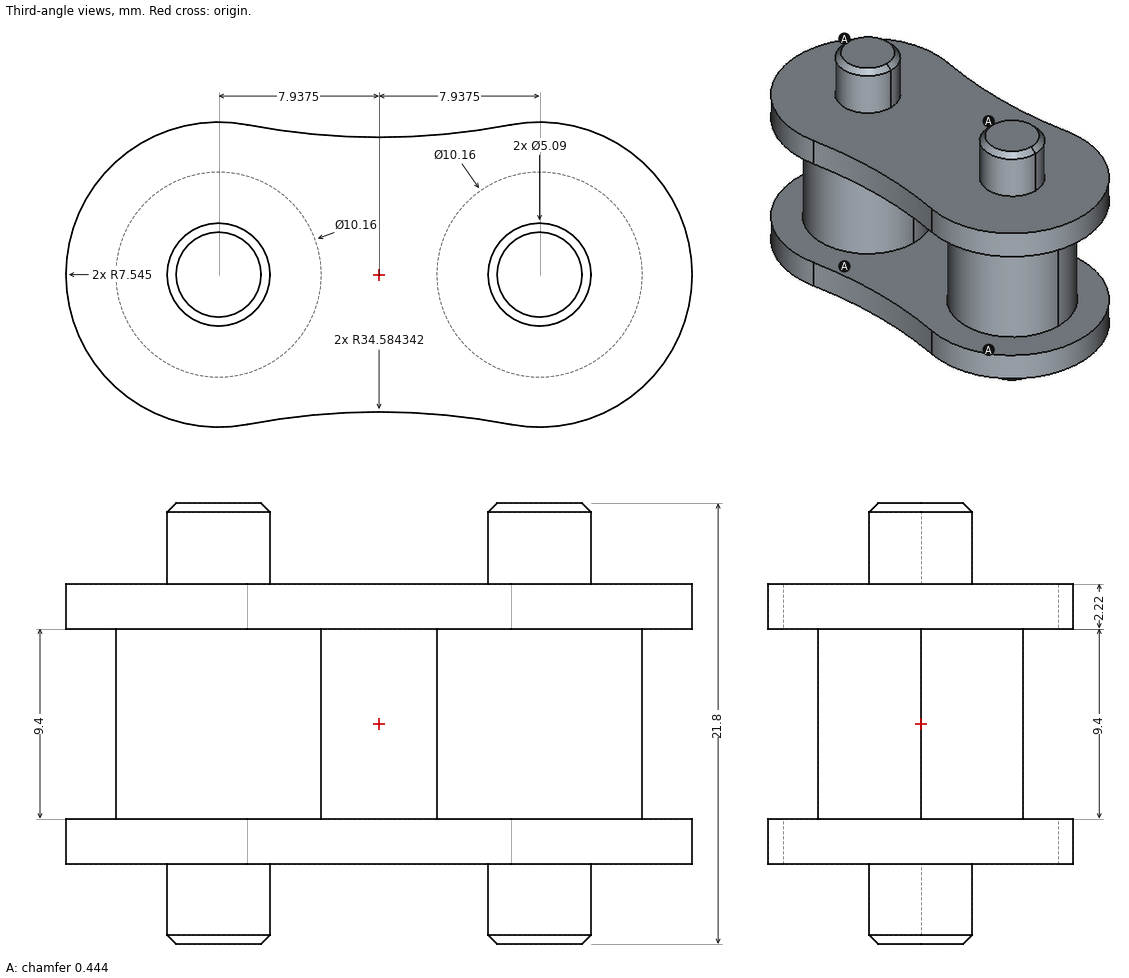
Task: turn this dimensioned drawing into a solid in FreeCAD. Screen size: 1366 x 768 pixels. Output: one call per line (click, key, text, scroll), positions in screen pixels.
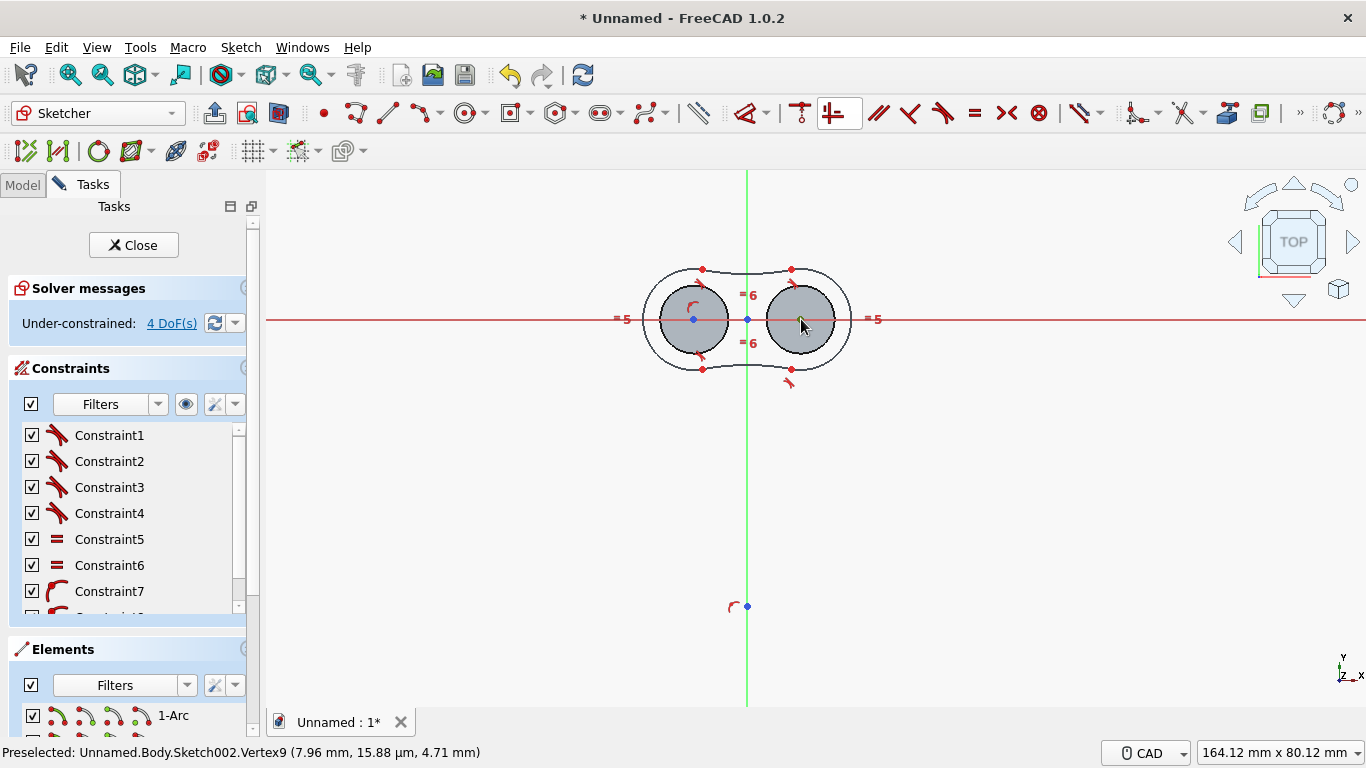
click(359, 320)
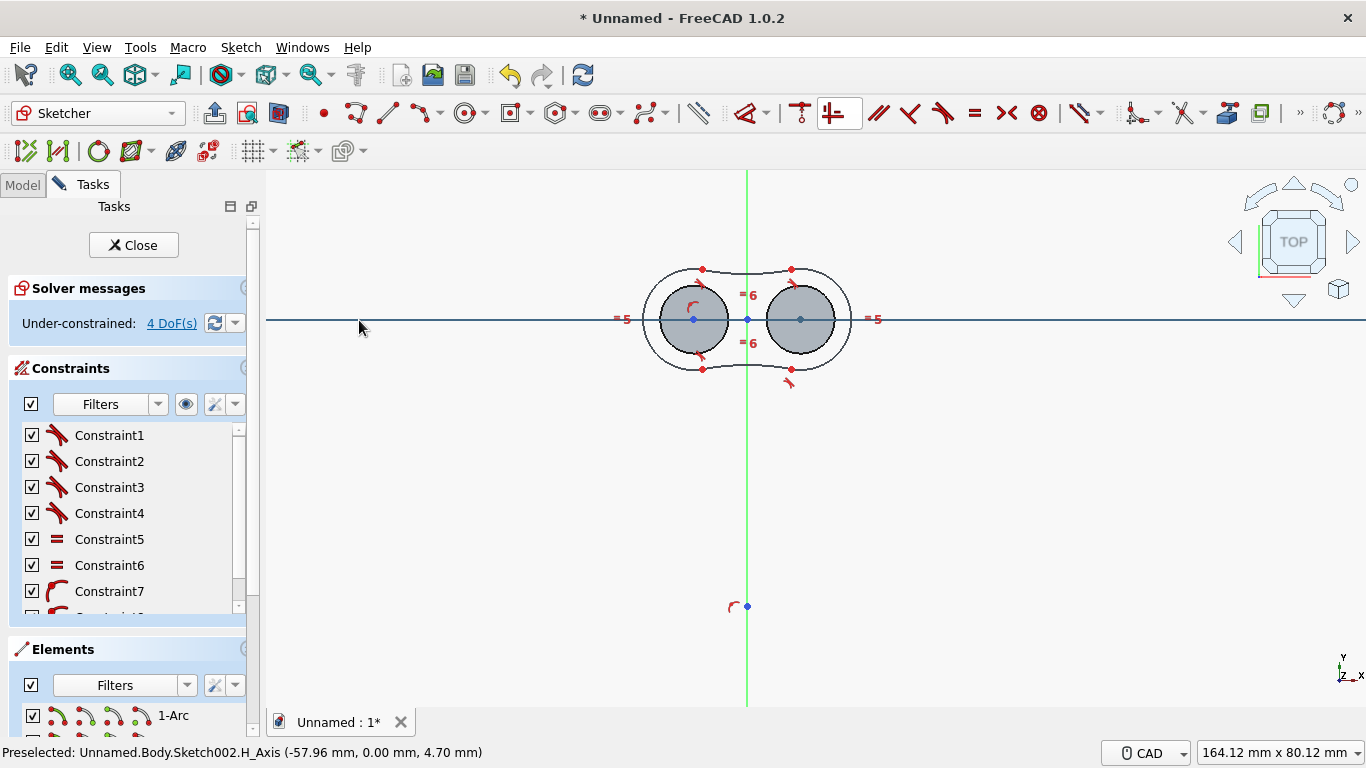
key(c)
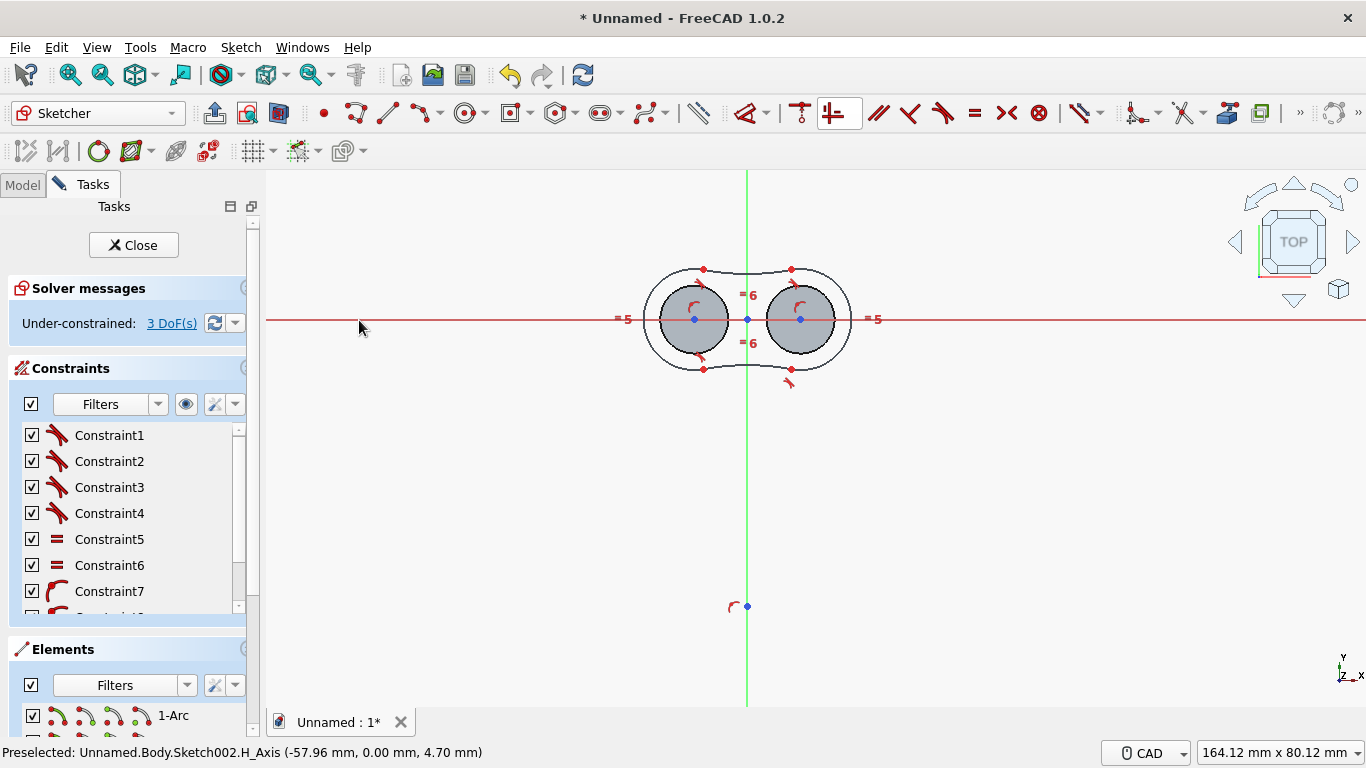
click(746, 114)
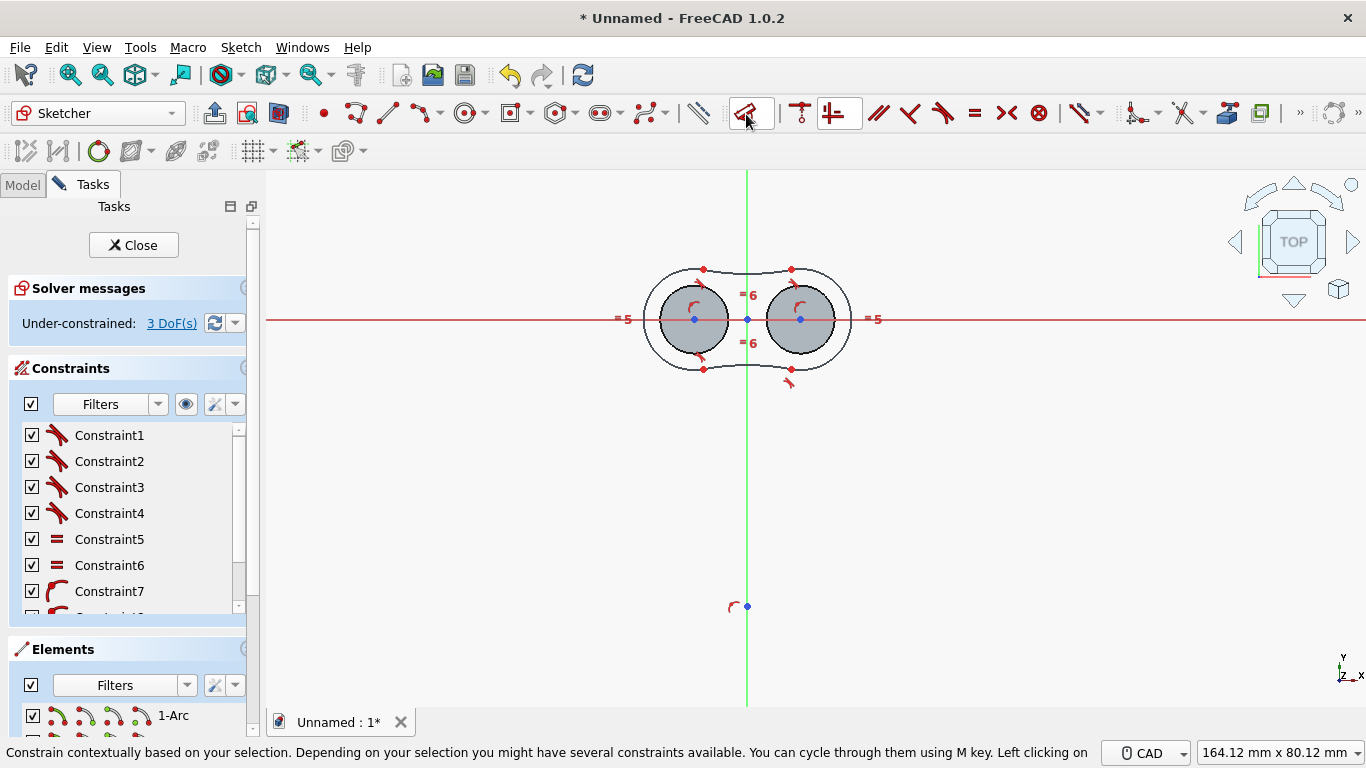
click(656, 287)
click(632, 266)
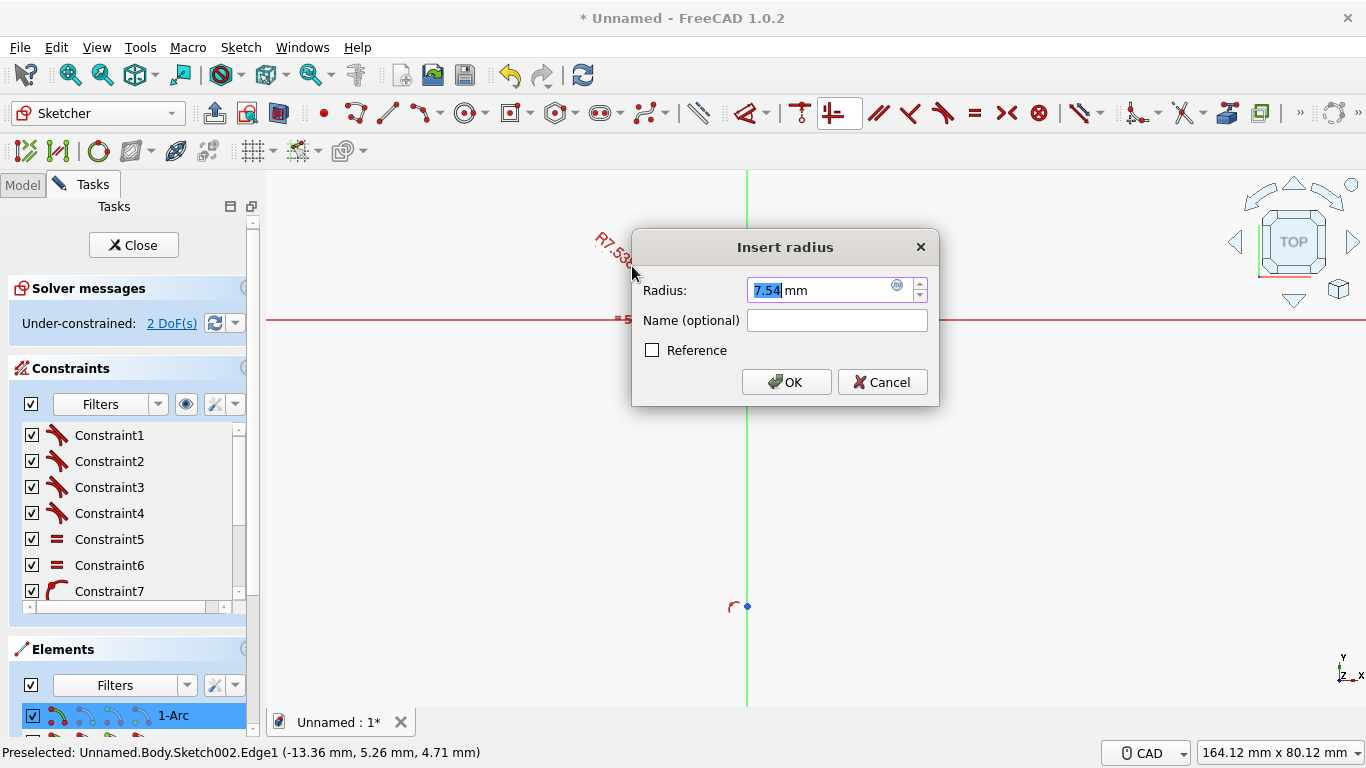
text(7.545)
key(Return)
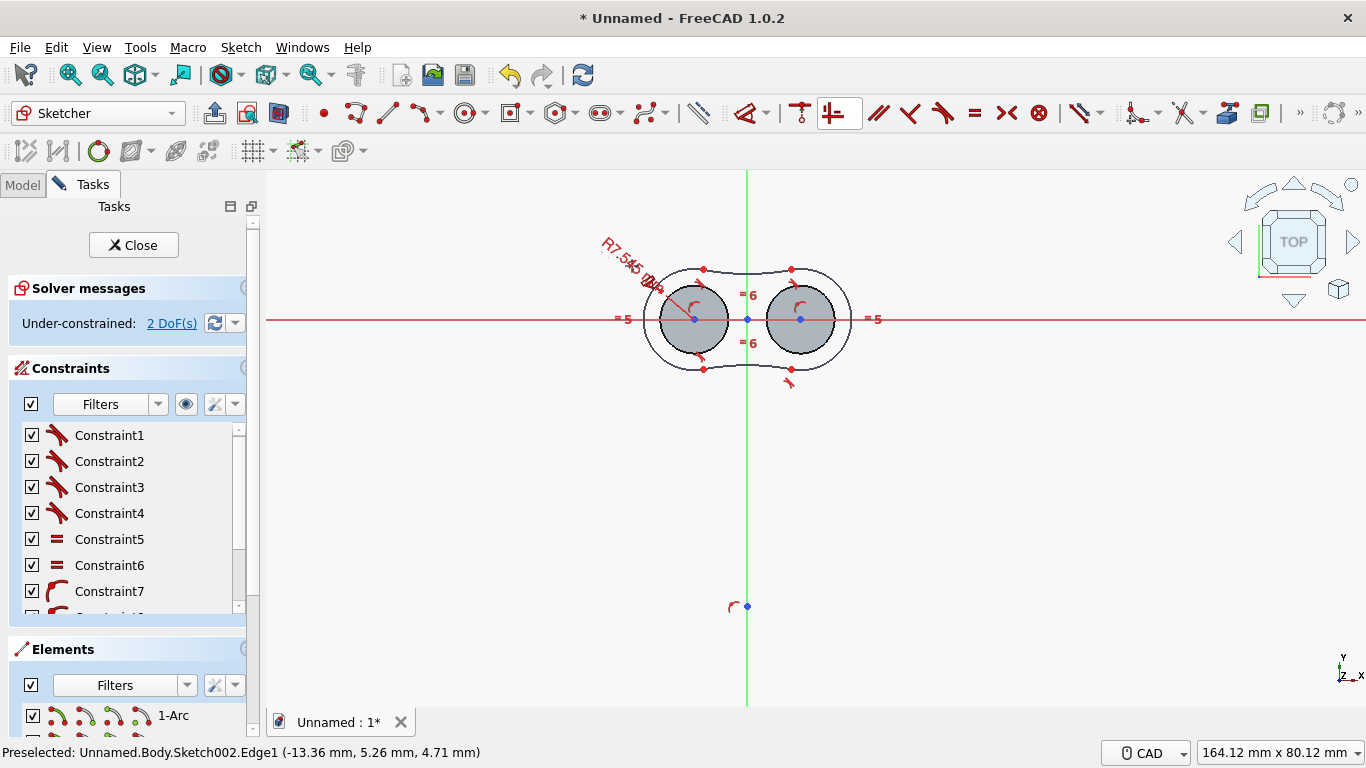
click(765, 366)
click(767, 334)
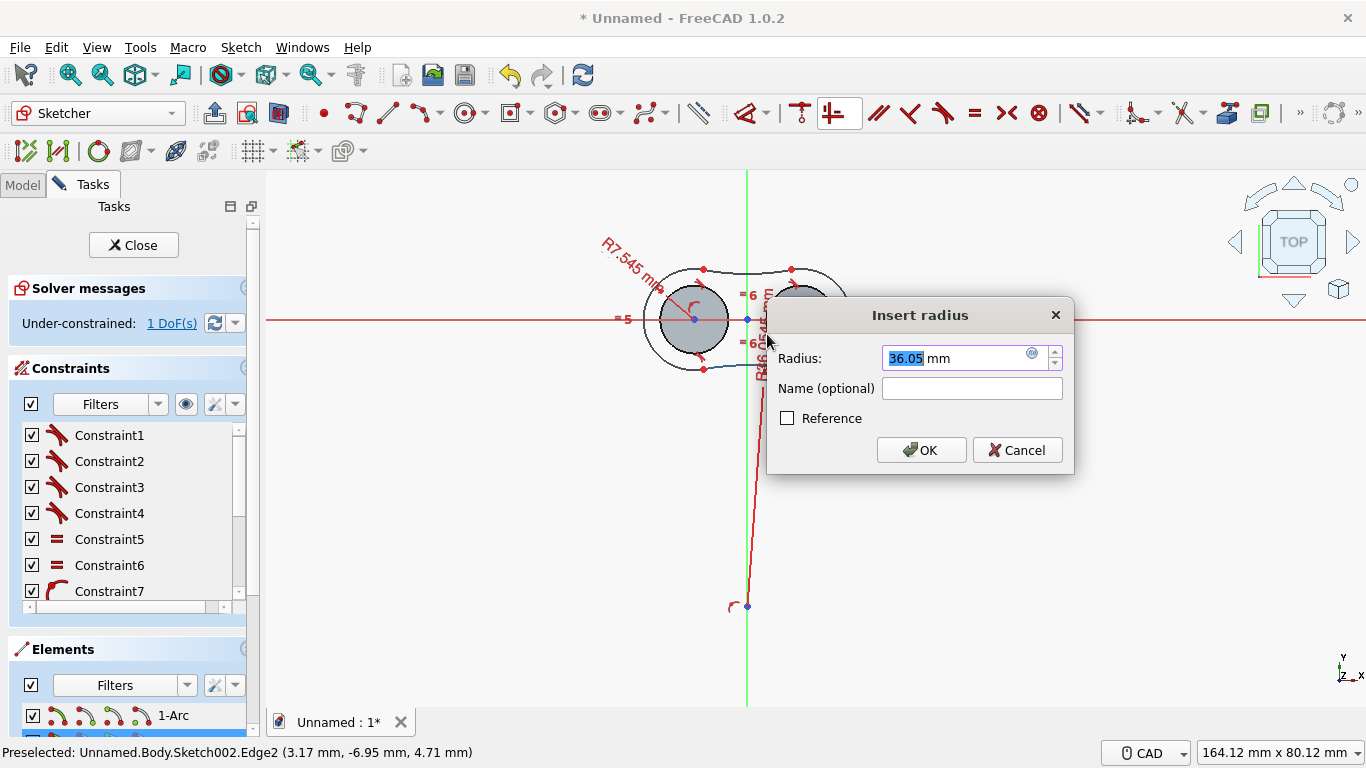
text(34.584342)
key(Return)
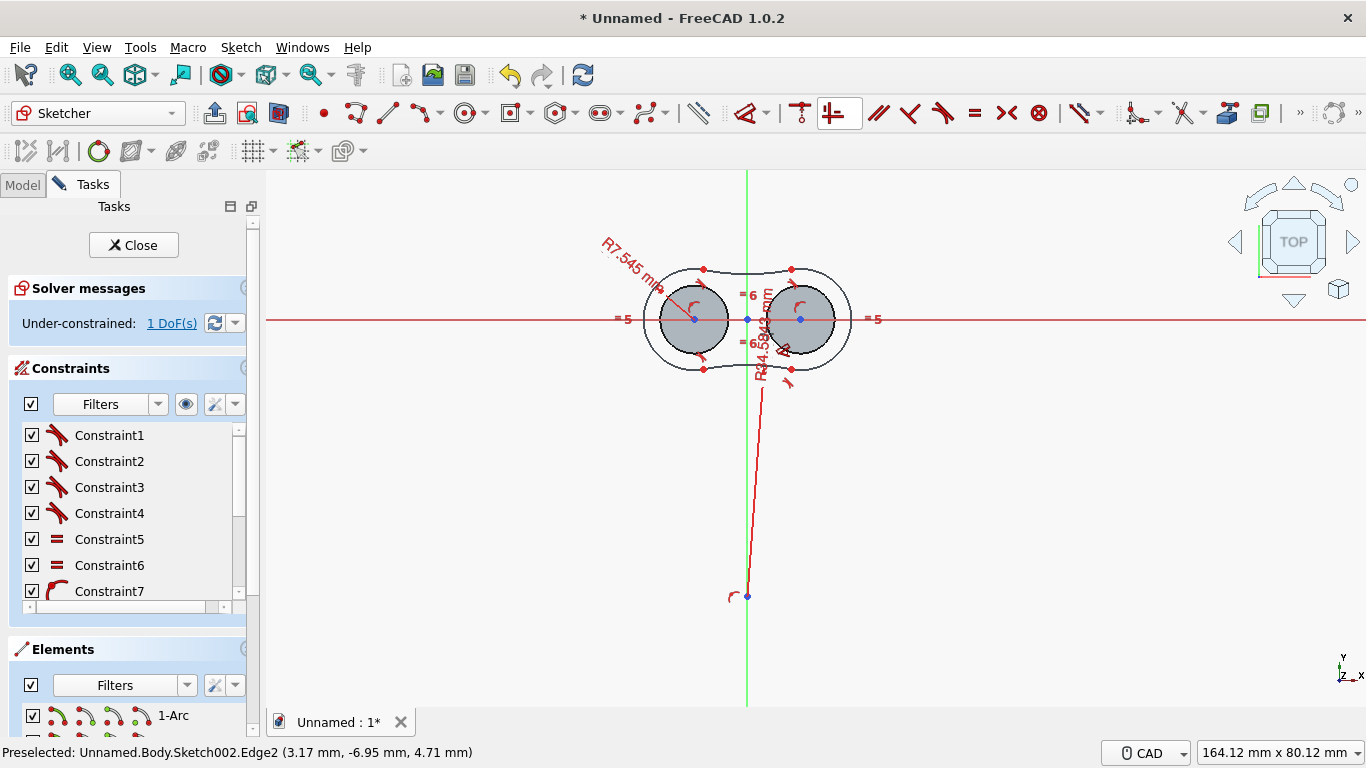
click(694, 320)
click(709, 286)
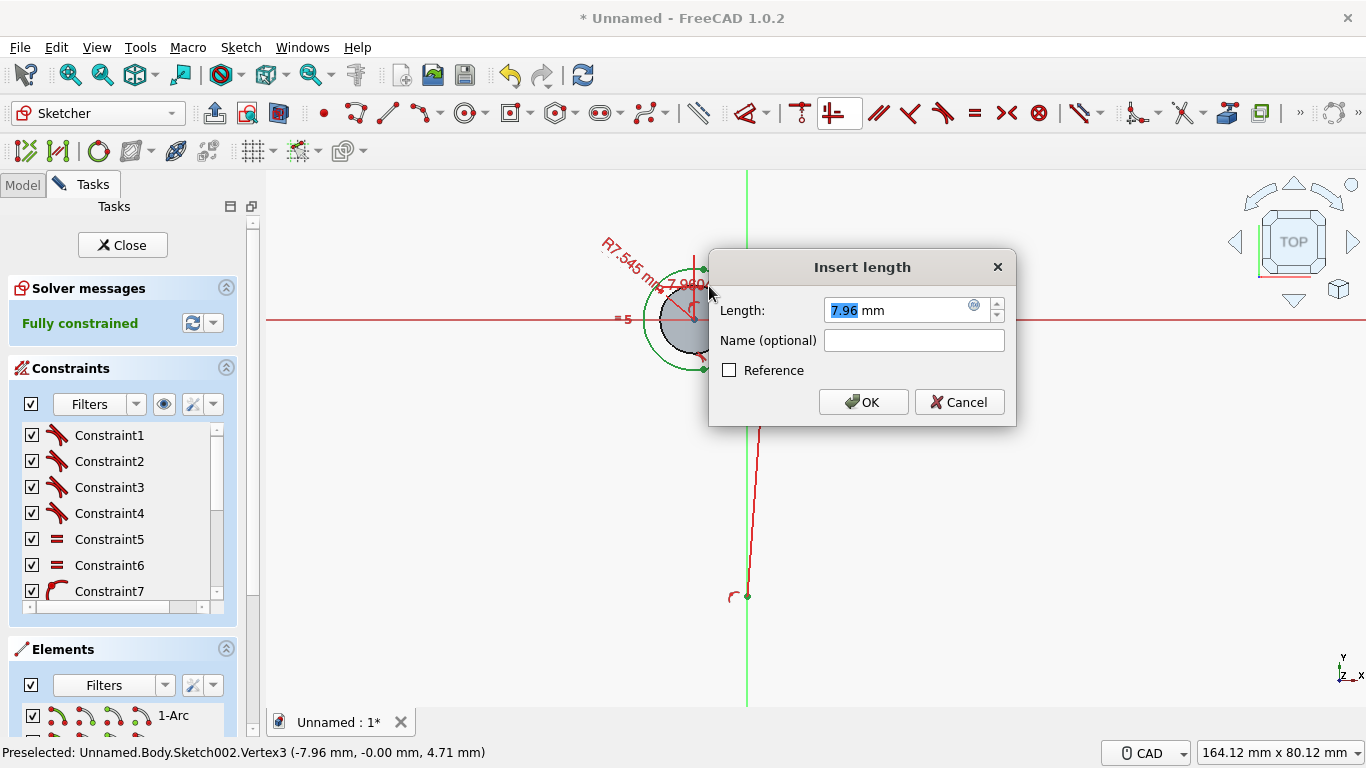
text(7.9375)
key(Return)
key(Escape)